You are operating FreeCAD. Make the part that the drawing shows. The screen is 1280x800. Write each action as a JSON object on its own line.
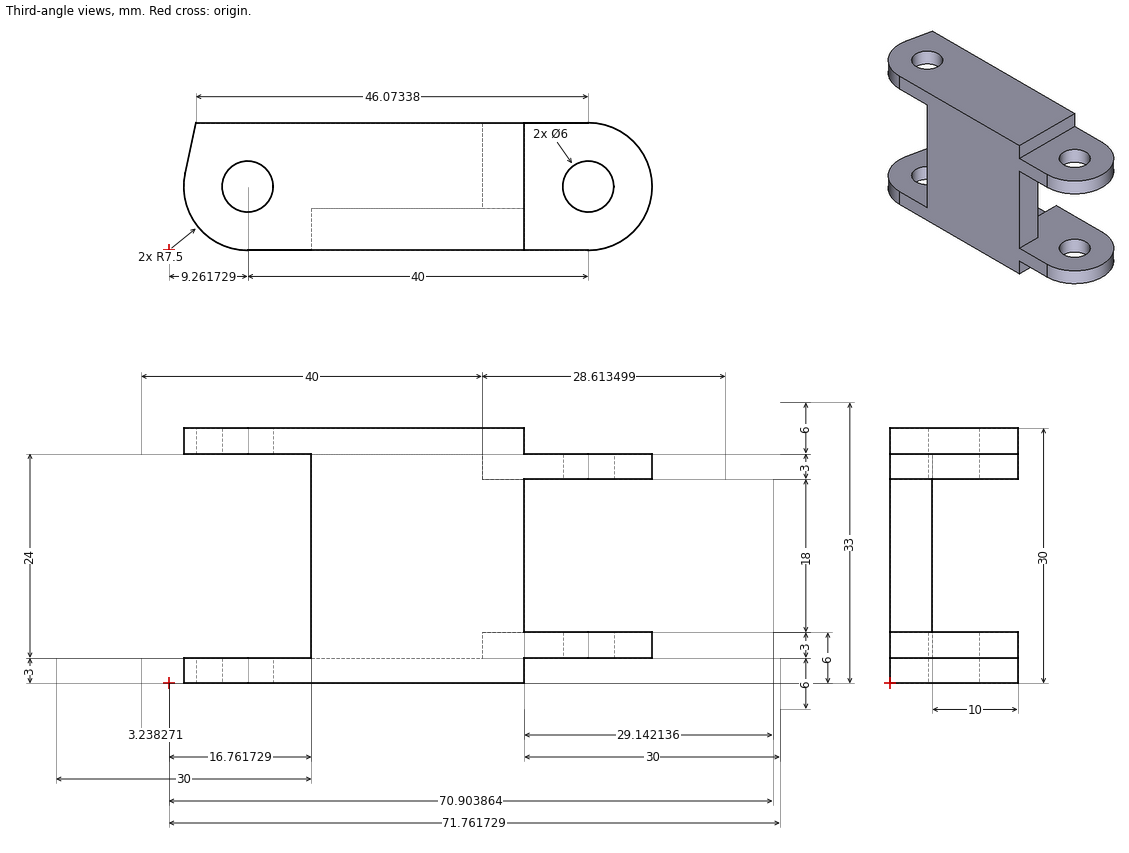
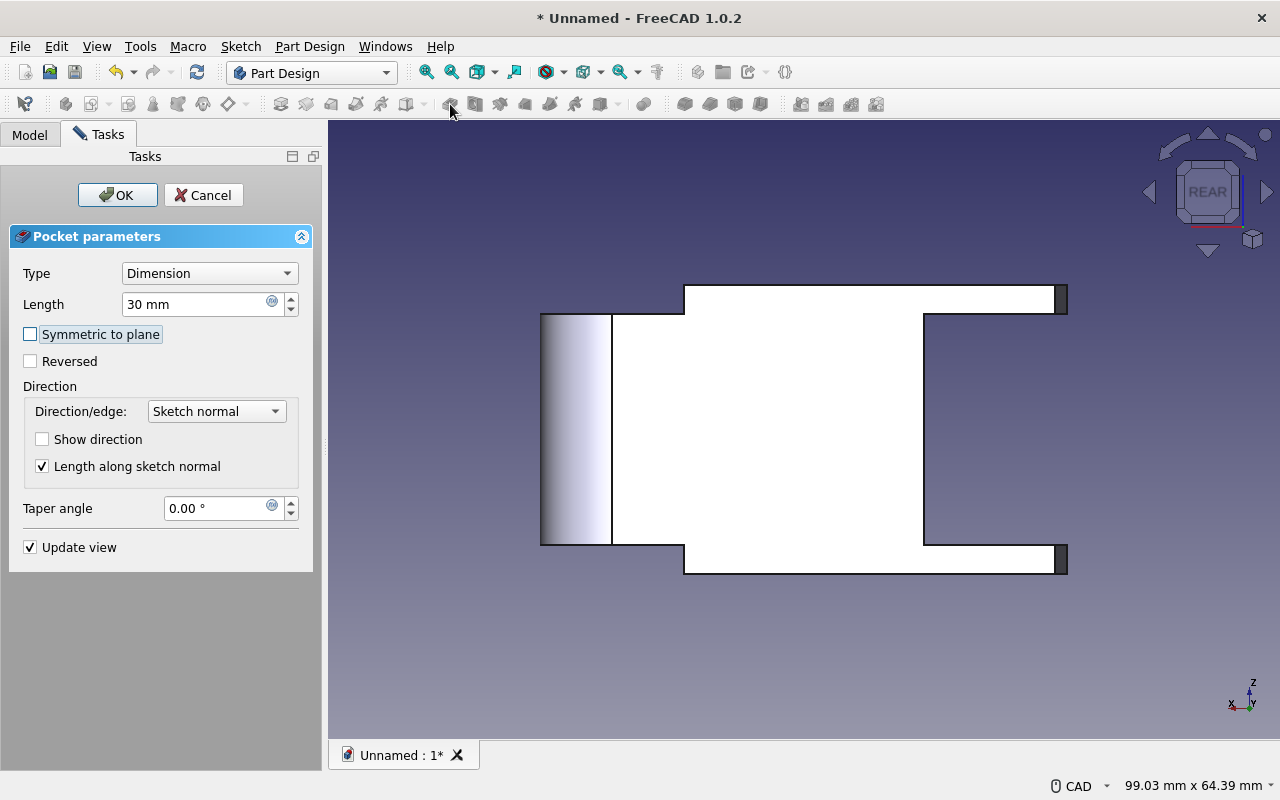
{"action": "left_click", "coordinate": [118, 195]}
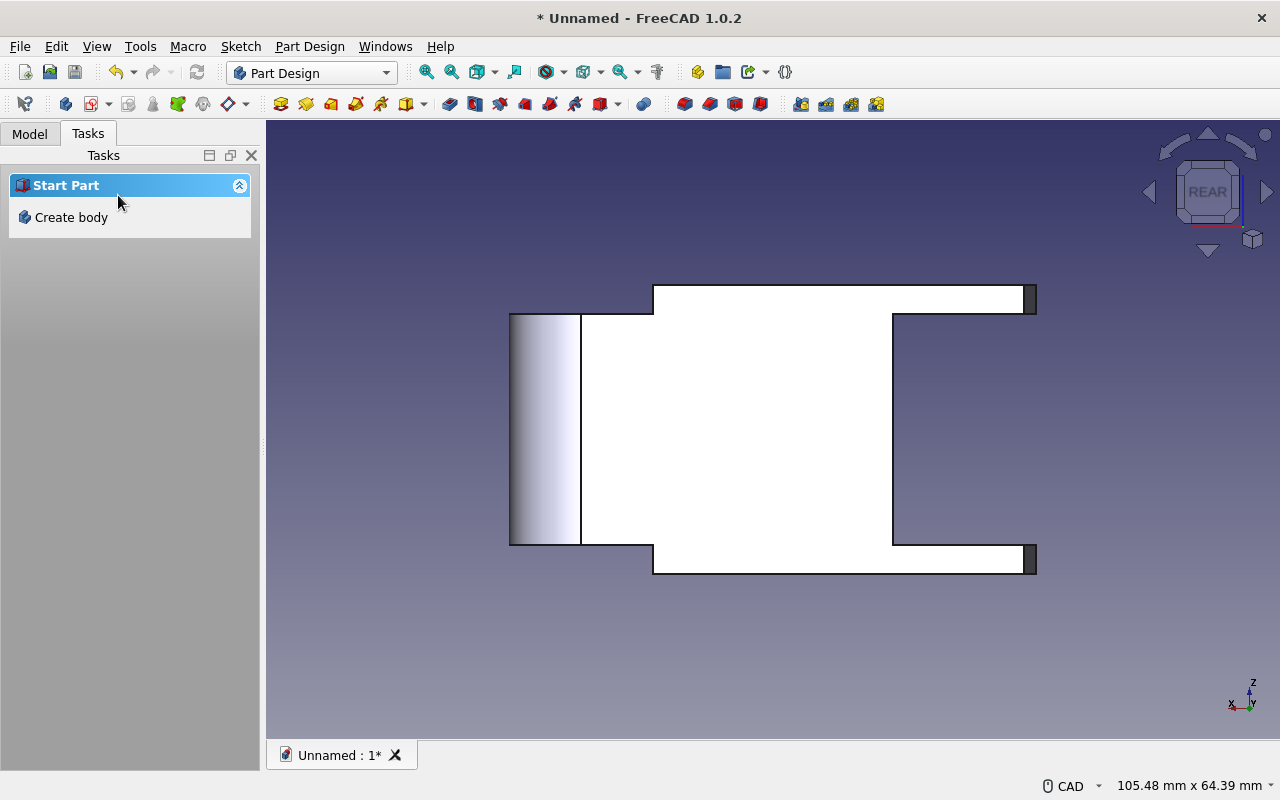
{"action": "left_click", "coordinate": [739, 429]}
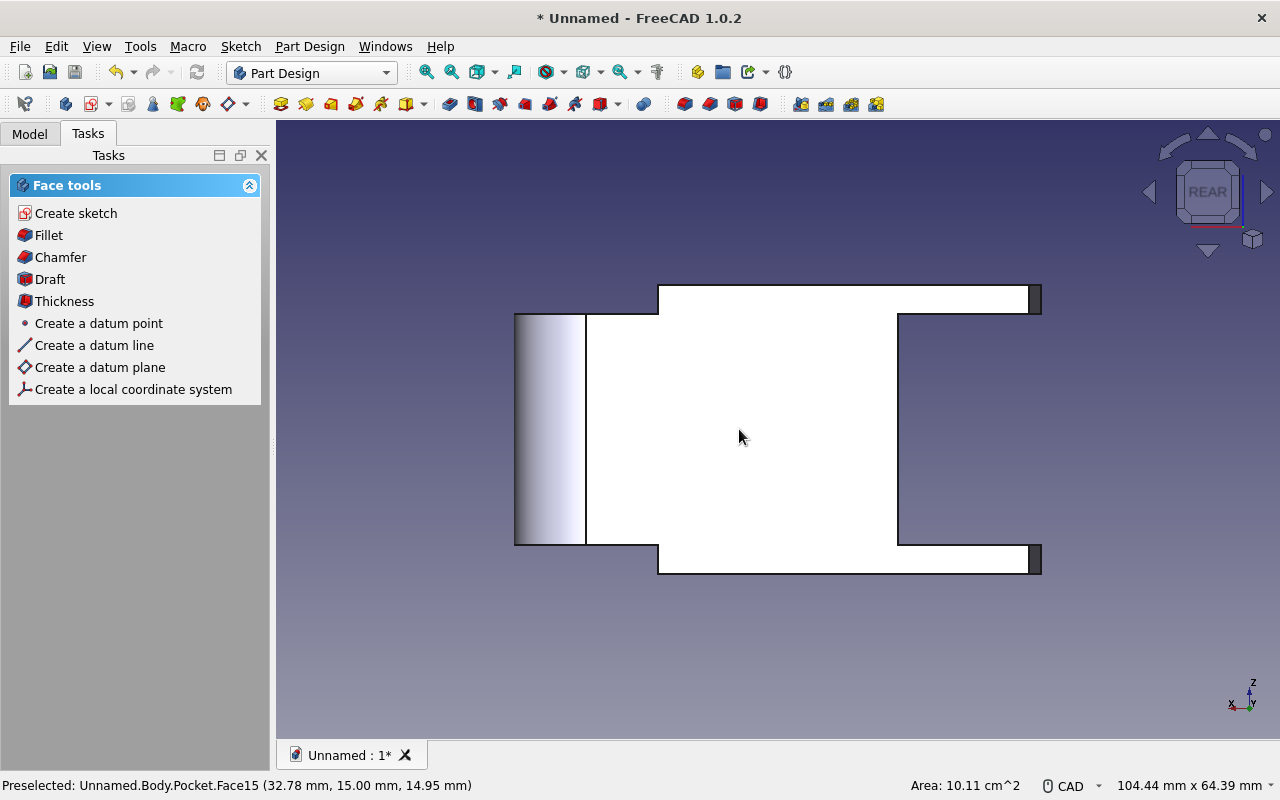
{"action": "left_click", "coordinate": [90, 104]}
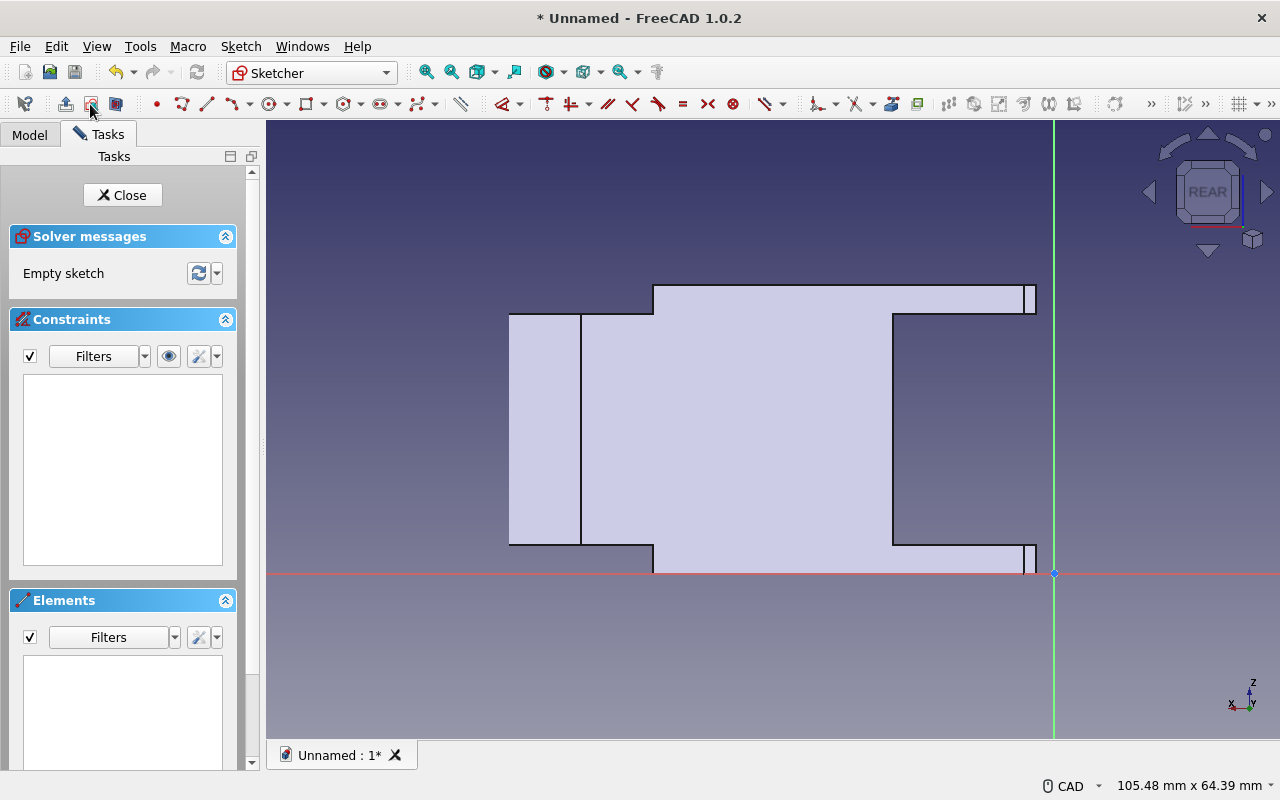
{"action": "left_click", "coordinate": [182, 104]}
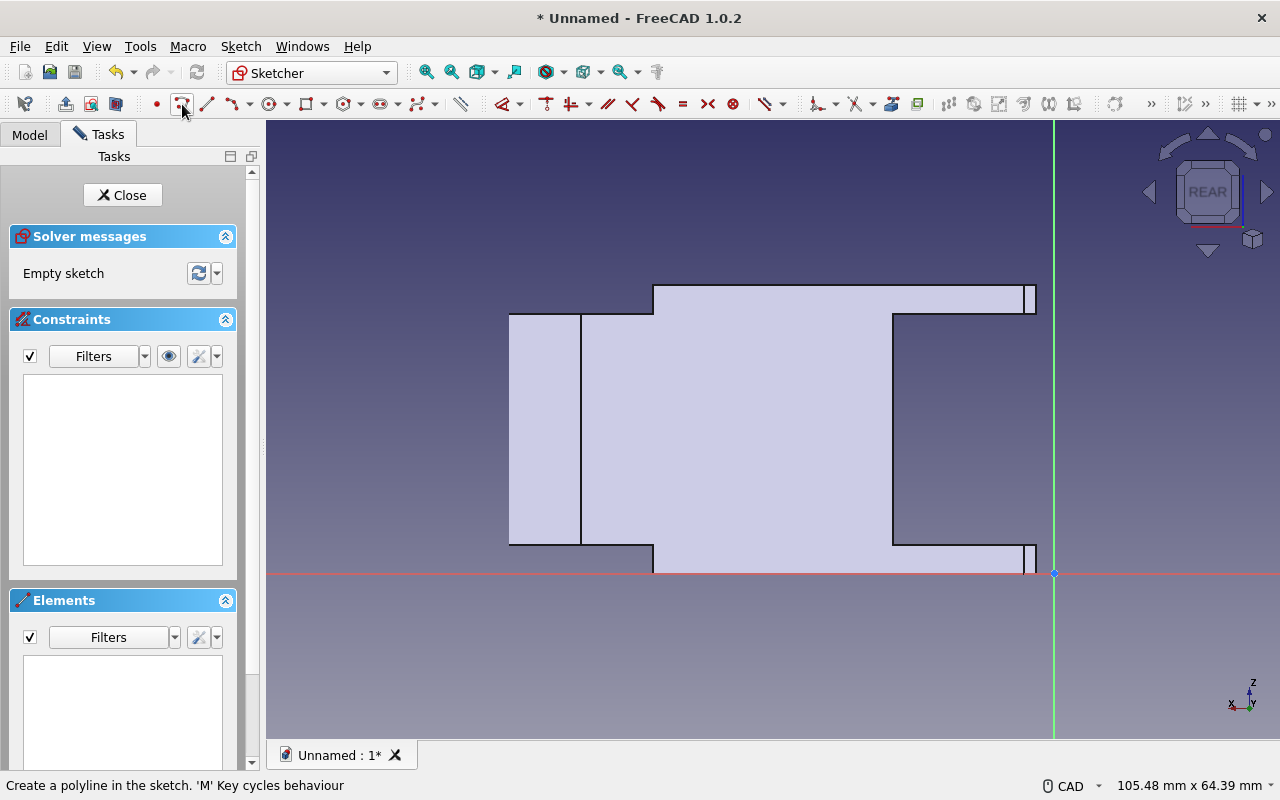
{"action": "left_click", "coordinate": [1085, 545]}
{"action": "left_click", "coordinate": [1085, 314]}
{"action": "left_click", "coordinate": [701, 314]}
{"action": "left_click", "coordinate": [701, 343]}
{"action": "left_click", "coordinate": [426, 343]}
{"action": "left_click", "coordinate": [426, 516]}
{"action": "left_click", "coordinate": [701, 516]}
{"action": "left_click", "coordinate": [701, 545]}
{"action": "left_click", "coordinate": [1085, 546]}
{"action": "key", "text": "Escape"}
{"action": "key", "text": "Escape"}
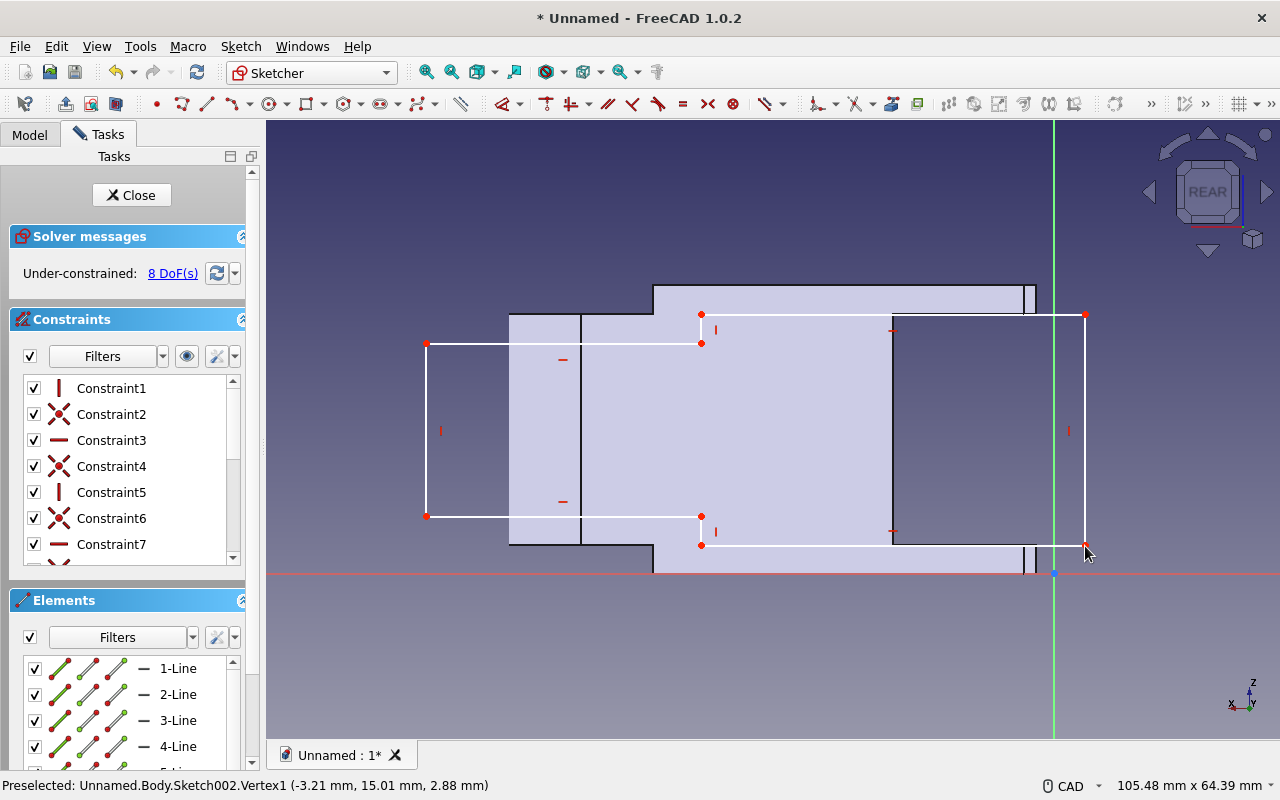
{"action": "key", "text": "d"}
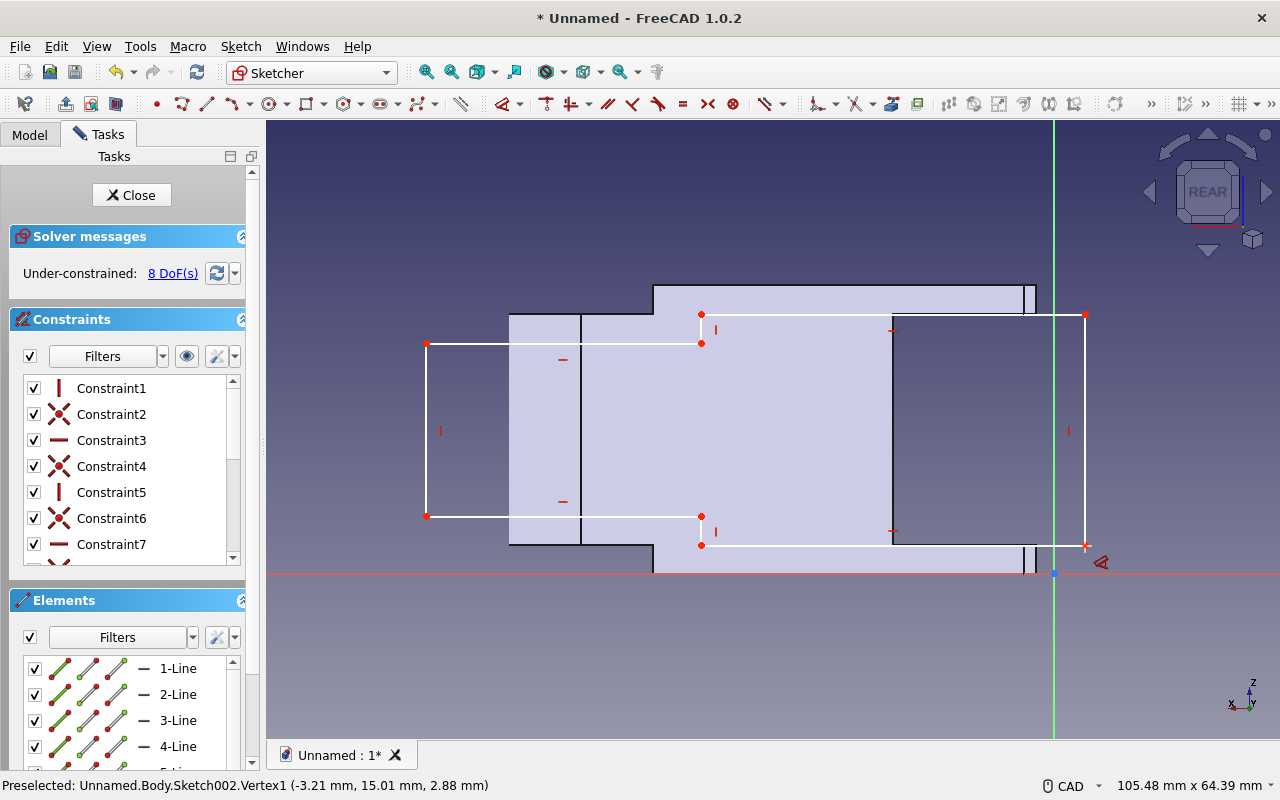
{"action": "scroll", "coordinate": [701, 327], "scroll_direction": "up", "scroll_amount": 2}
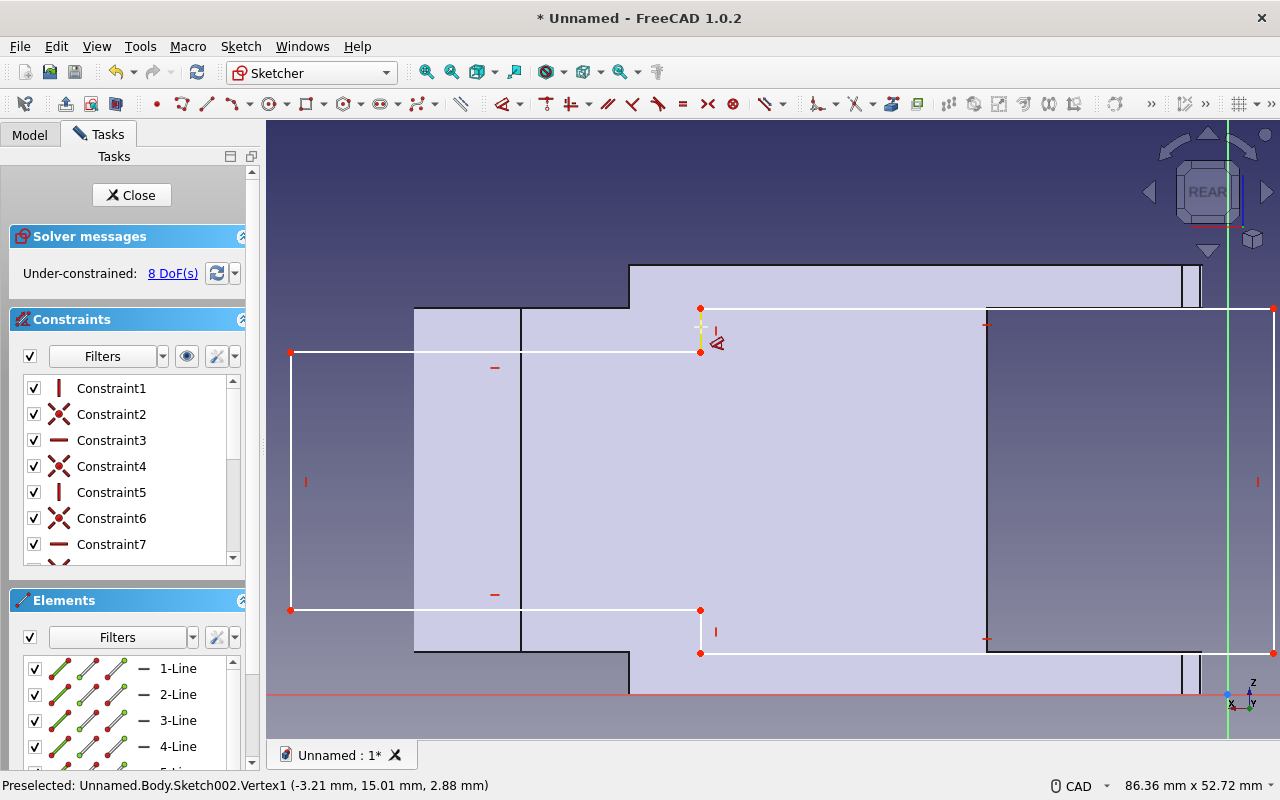
{"action": "left_click", "coordinate": [701, 326]}
{"action": "left_click", "coordinate": [667, 331]}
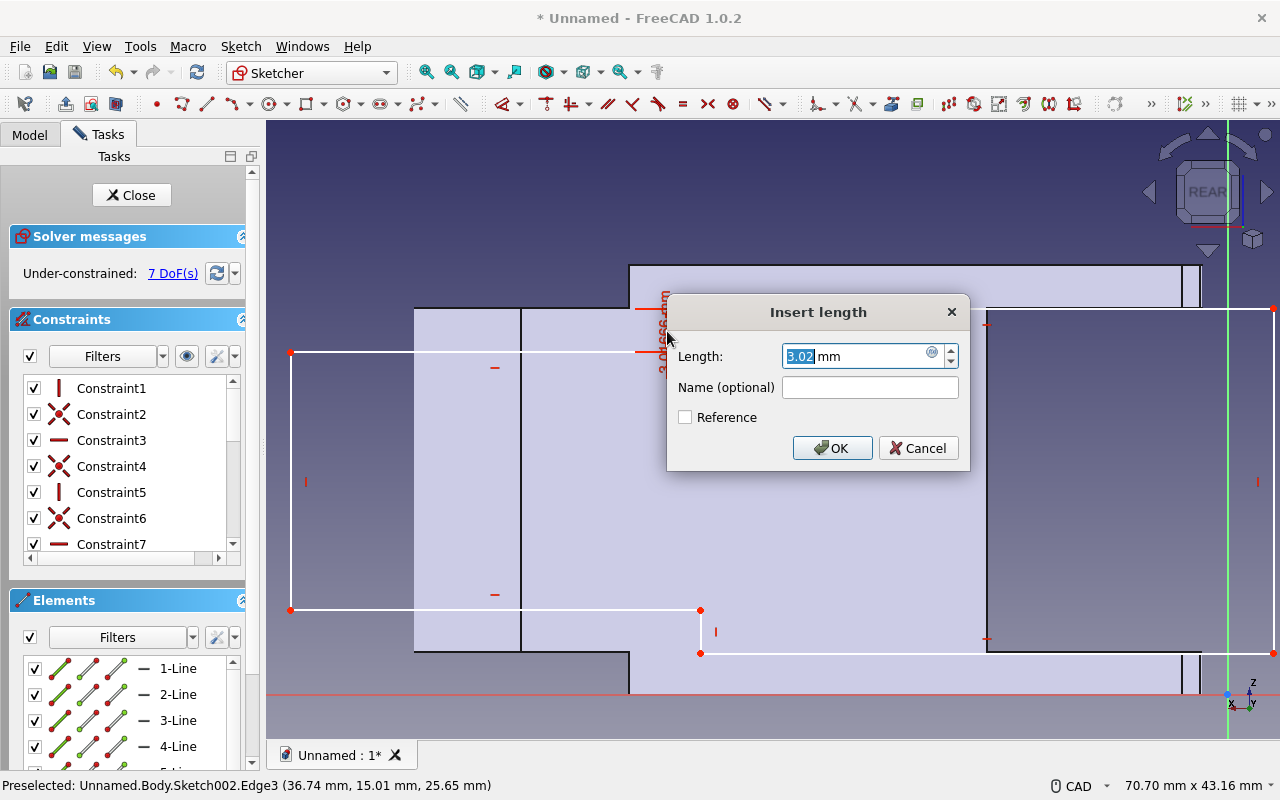
{"action": "type", "text": "3"}
{"action": "key", "text": "Return"}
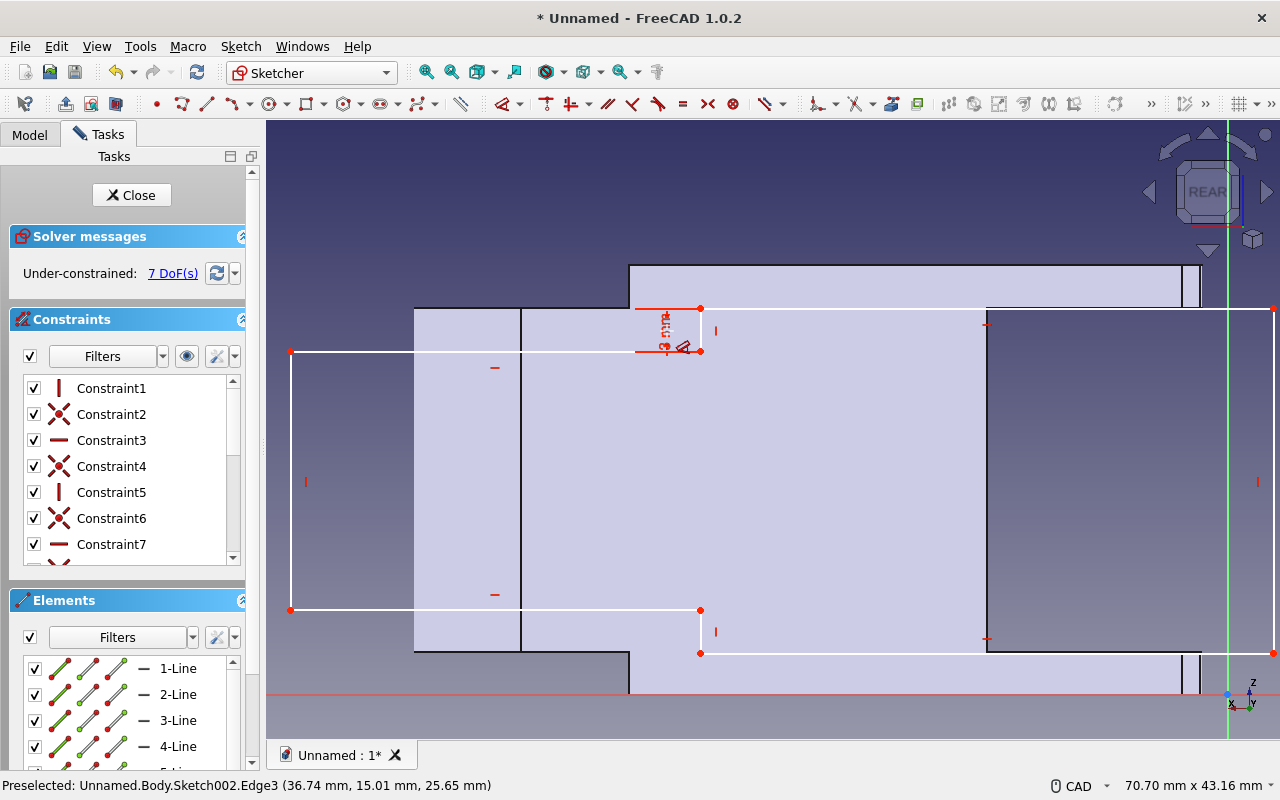
{"action": "left_click", "coordinate": [701, 623]}
{"action": "left_click", "coordinate": [667, 632]}